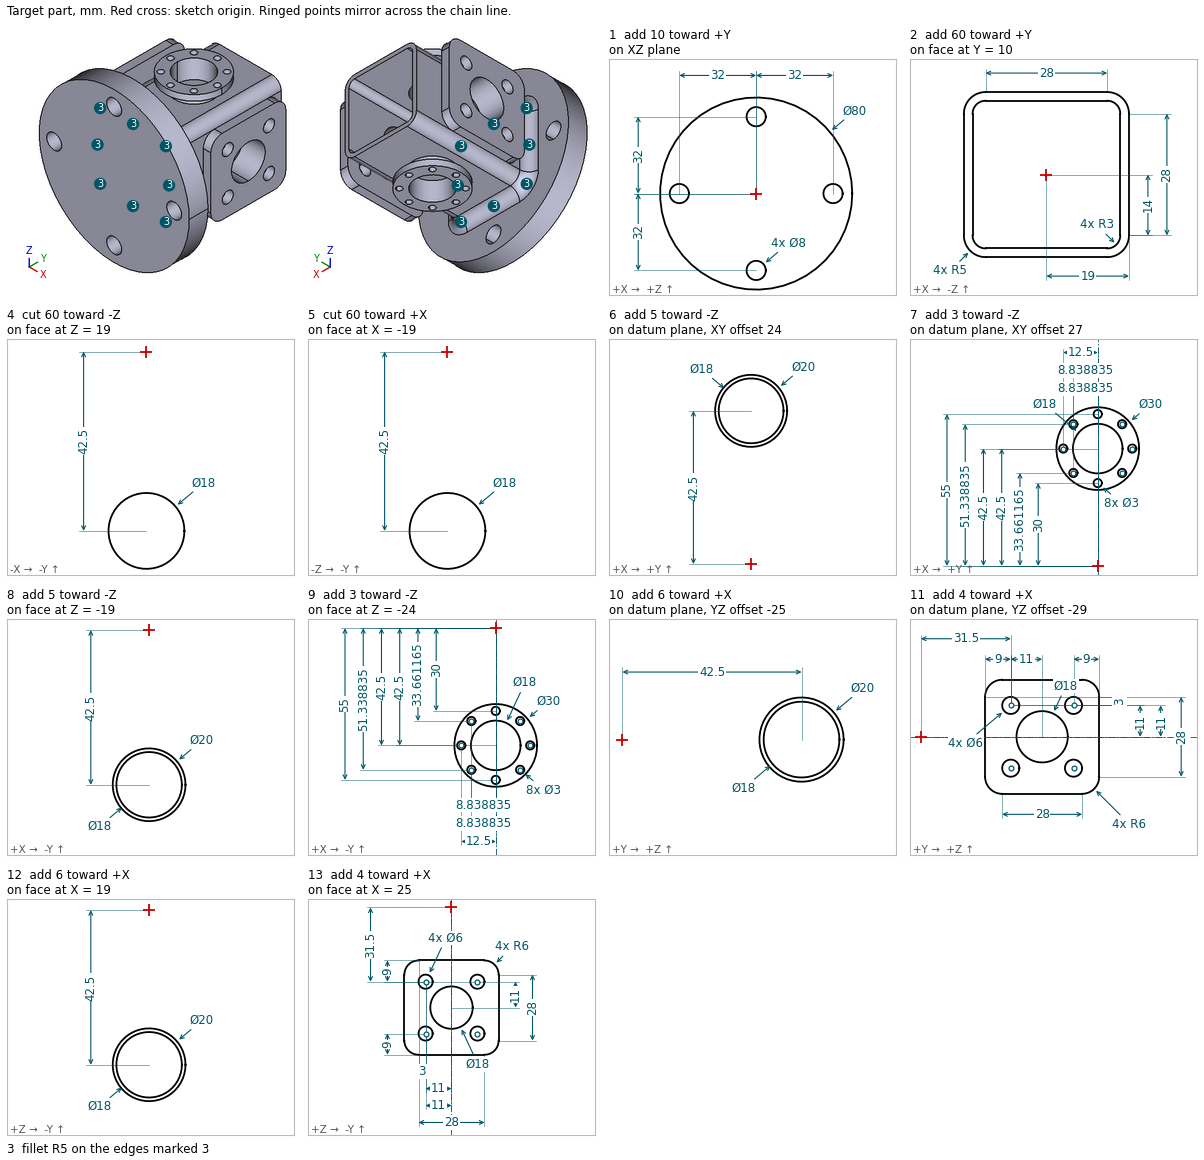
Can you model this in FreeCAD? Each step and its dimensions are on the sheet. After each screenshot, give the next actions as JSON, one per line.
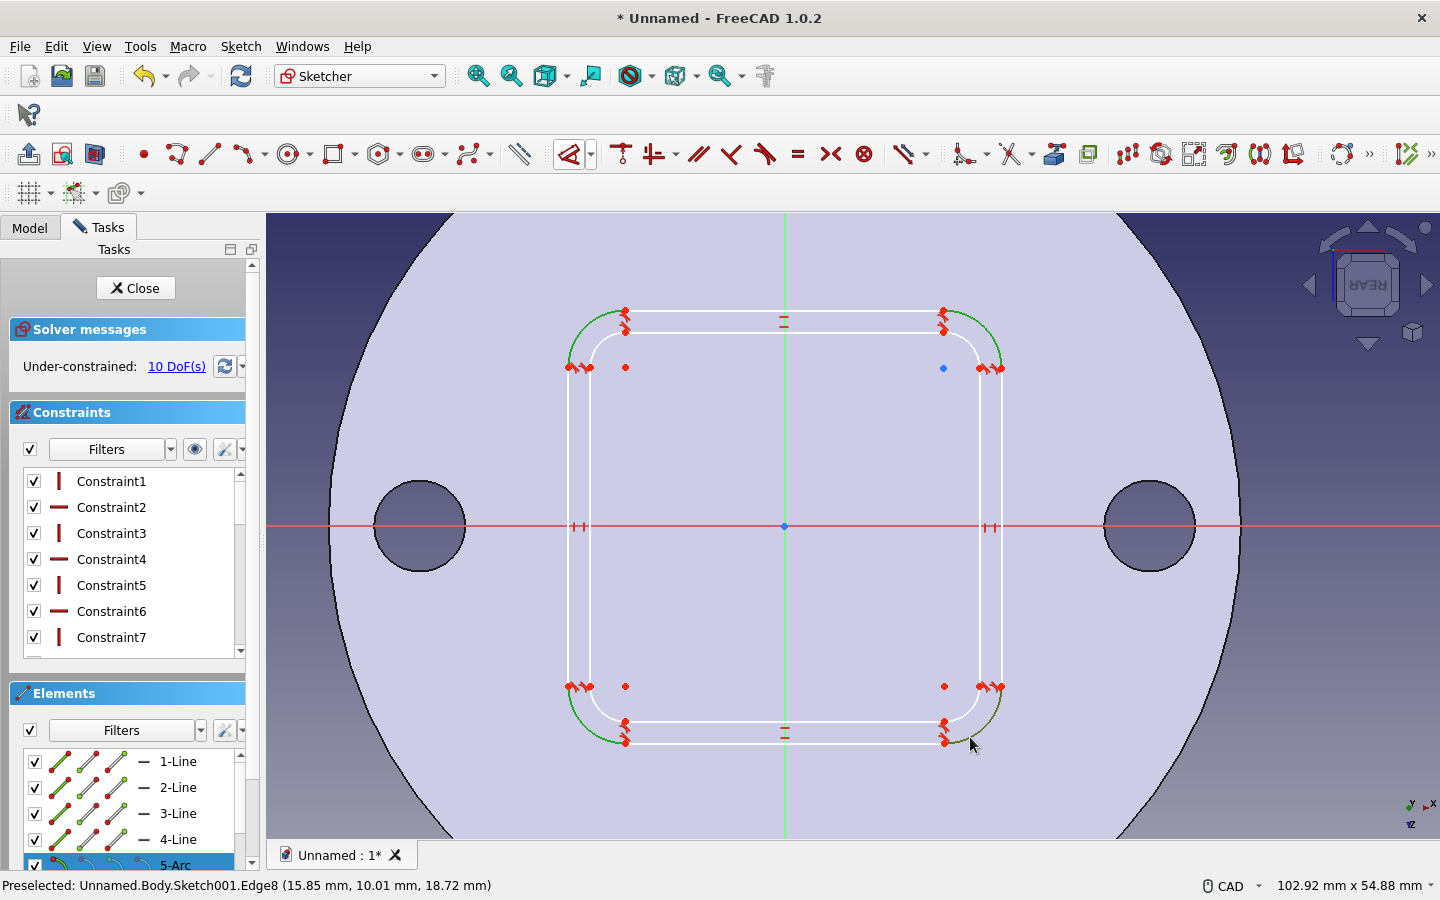
{"action": "key", "text": "e"}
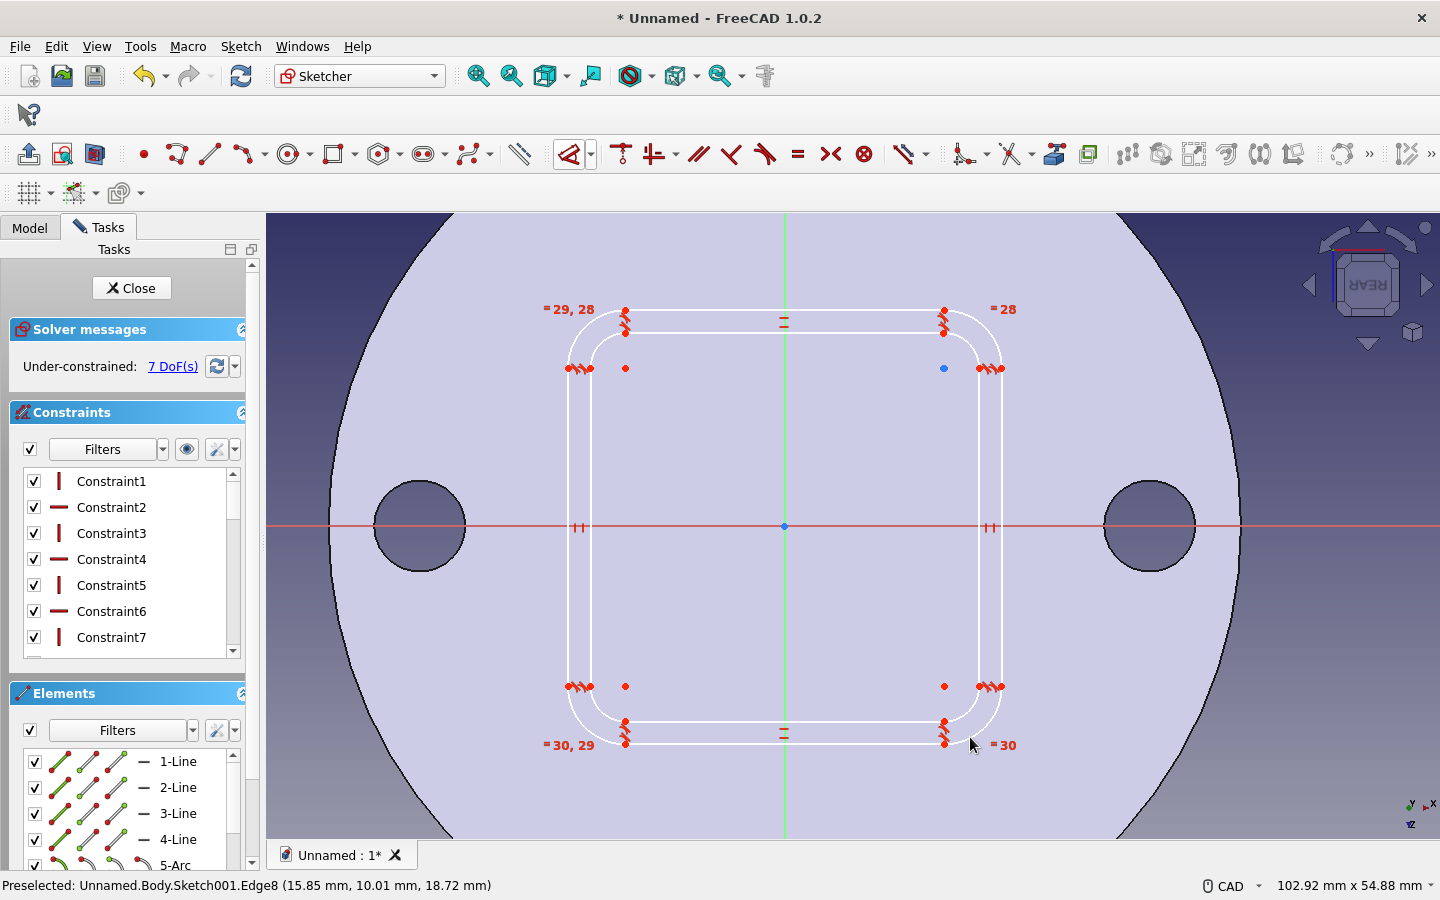
{"action": "left_click", "coordinate": [960, 718]}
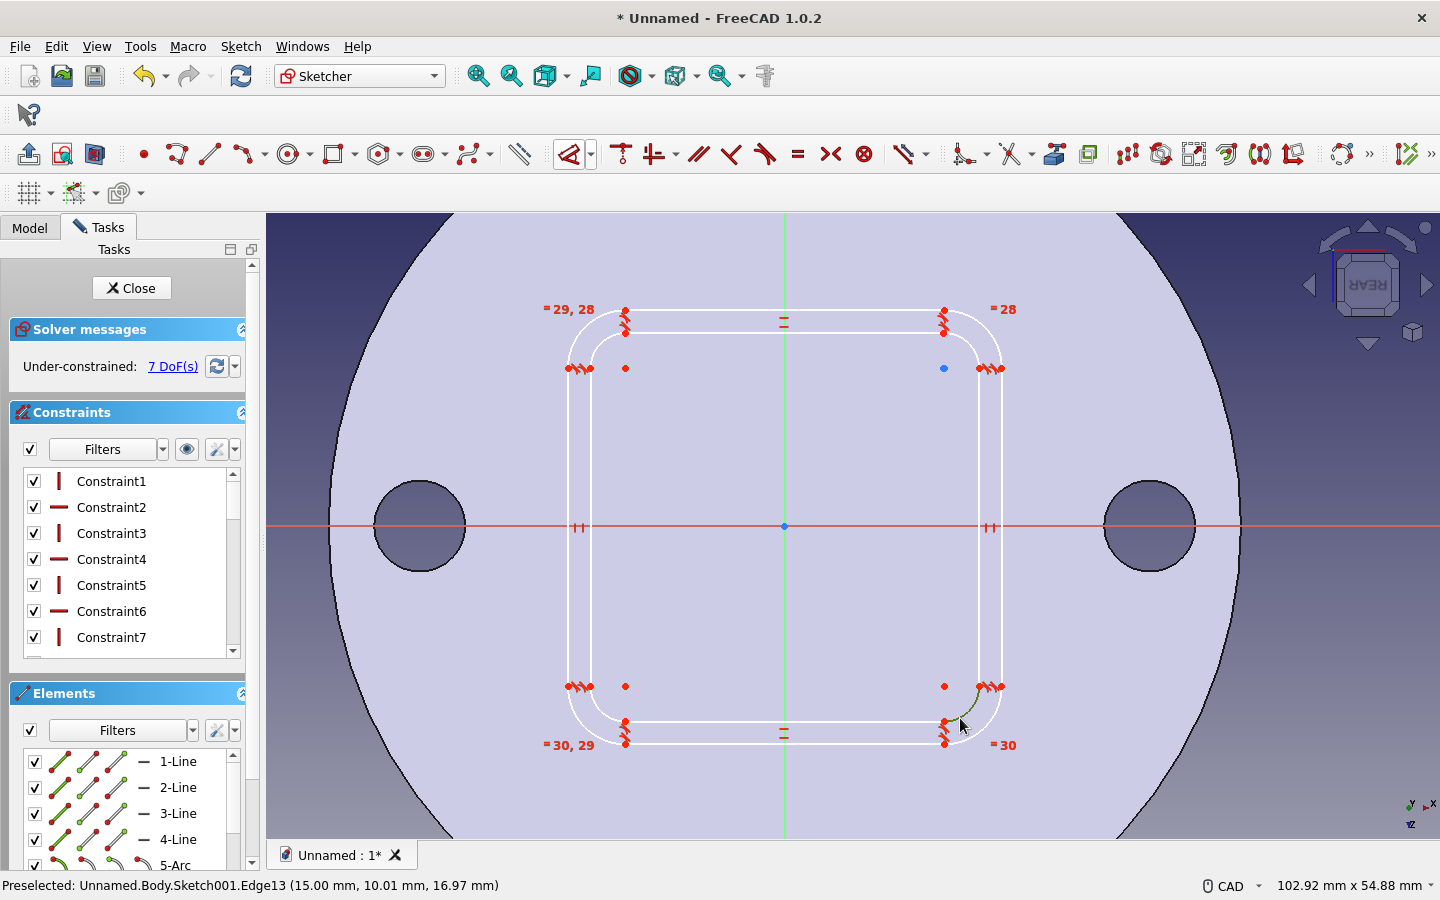
{"action": "left_click", "coordinate": [975, 352]}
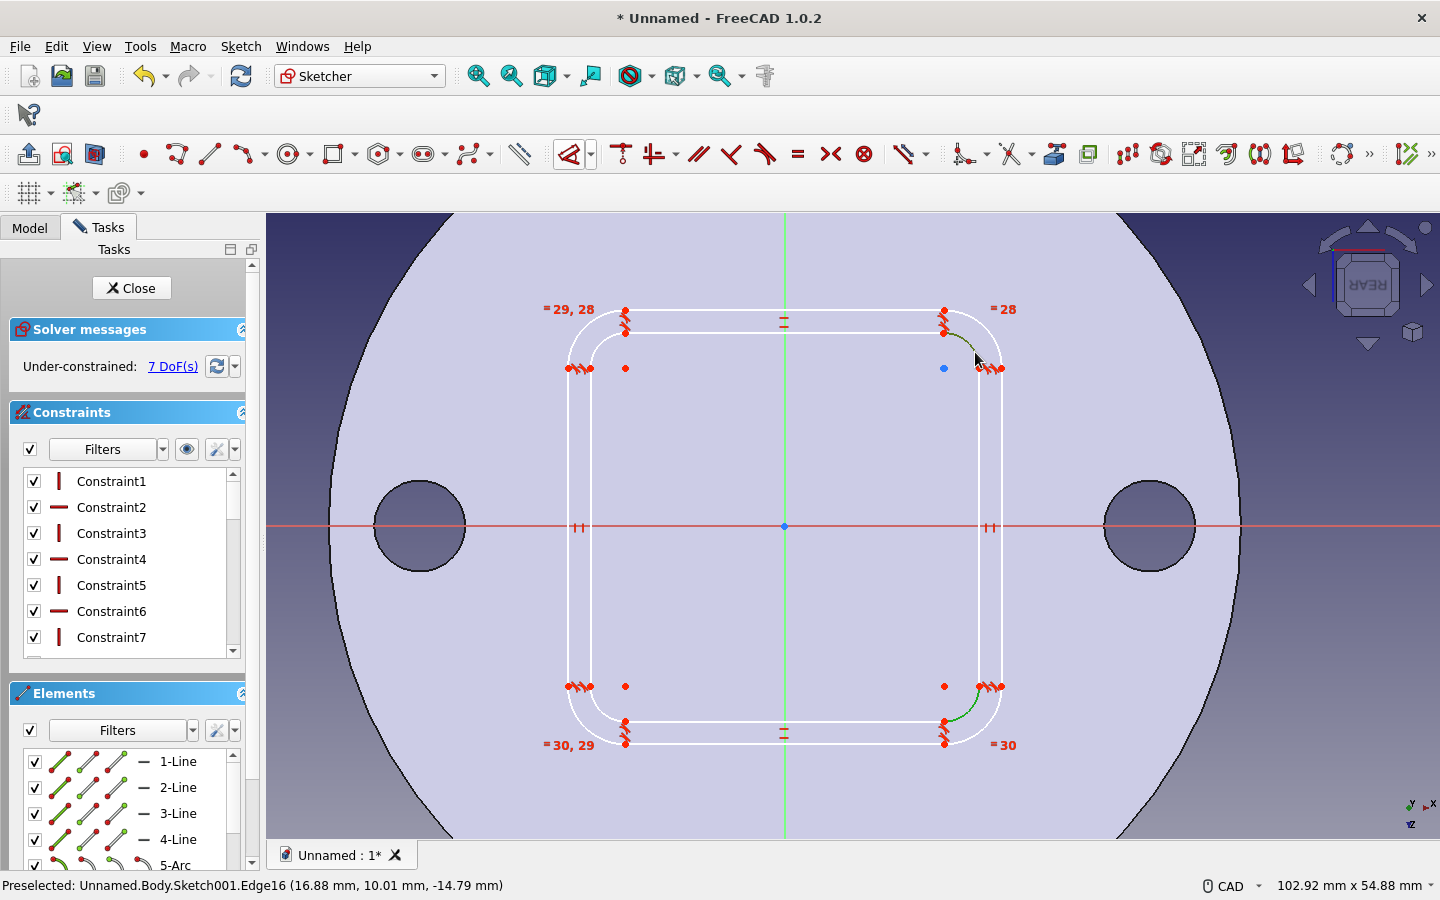
{"action": "key", "text": "e"}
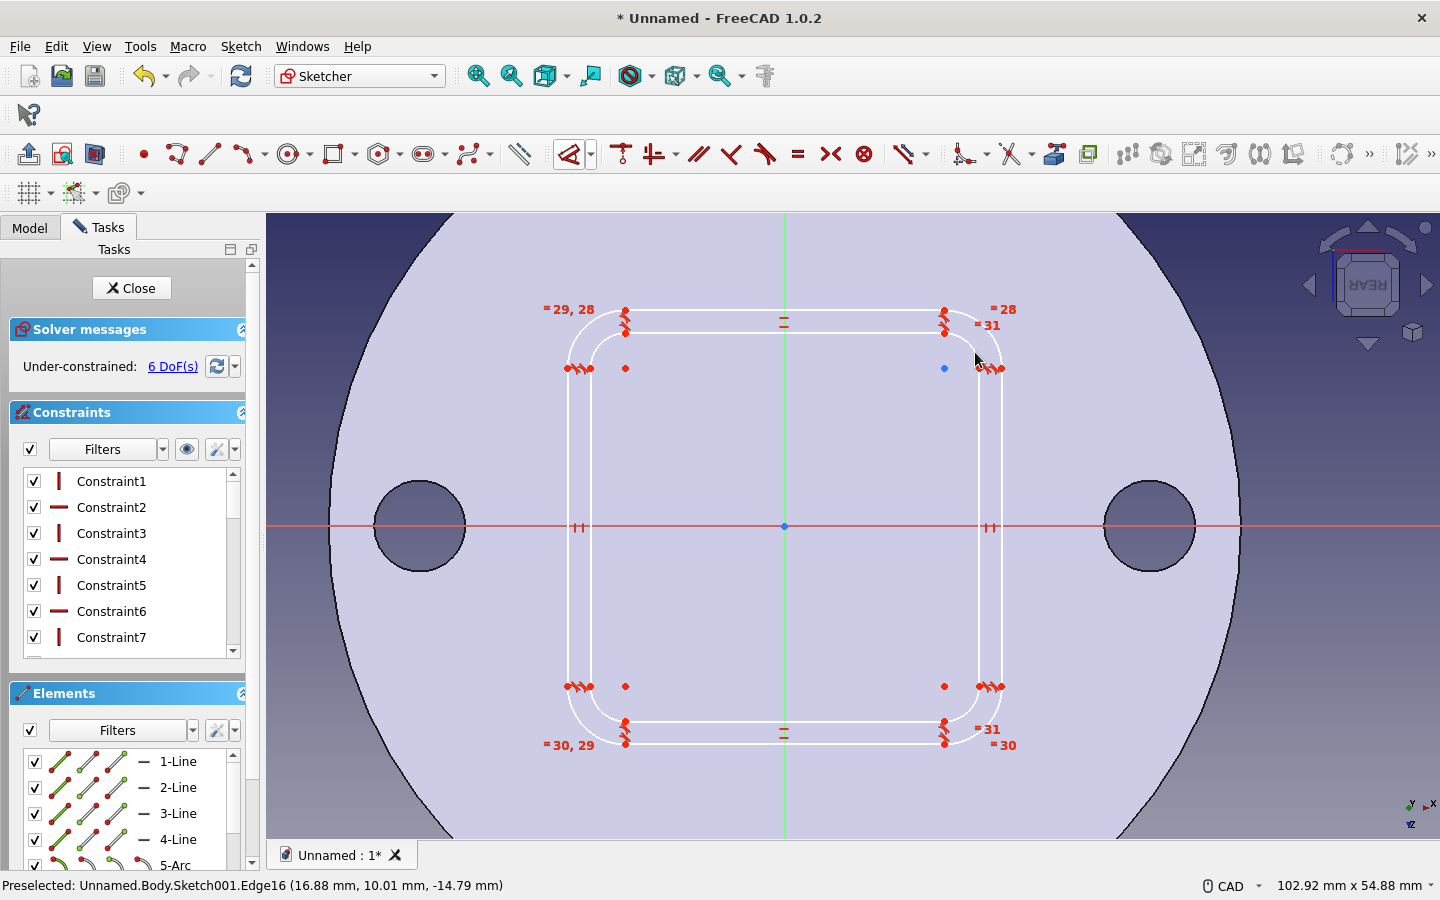
{"action": "left_click", "coordinate": [996, 342]}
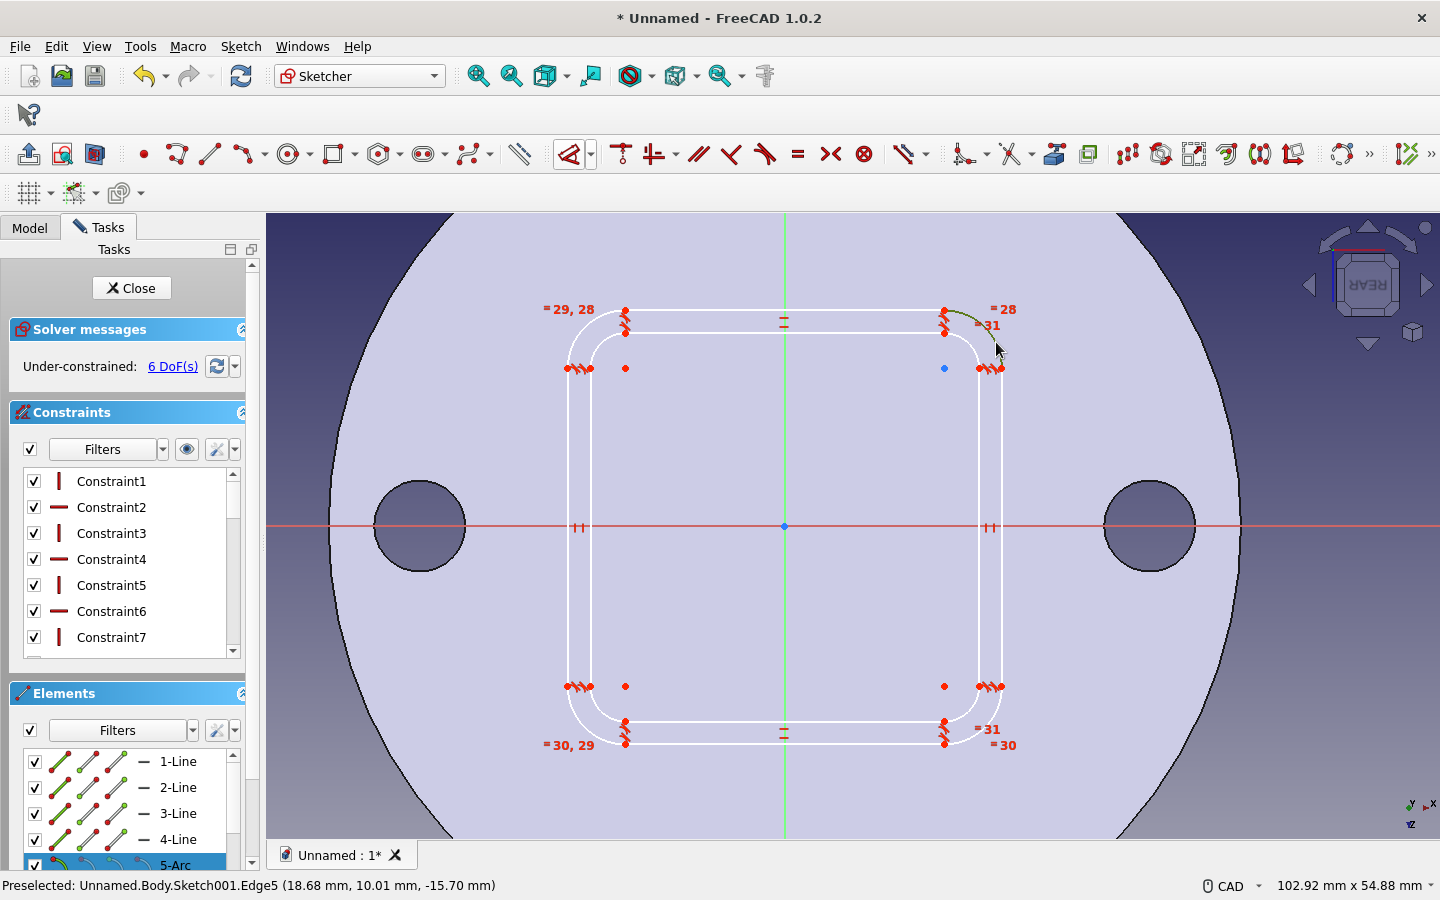
{"action": "key", "text": "k r"}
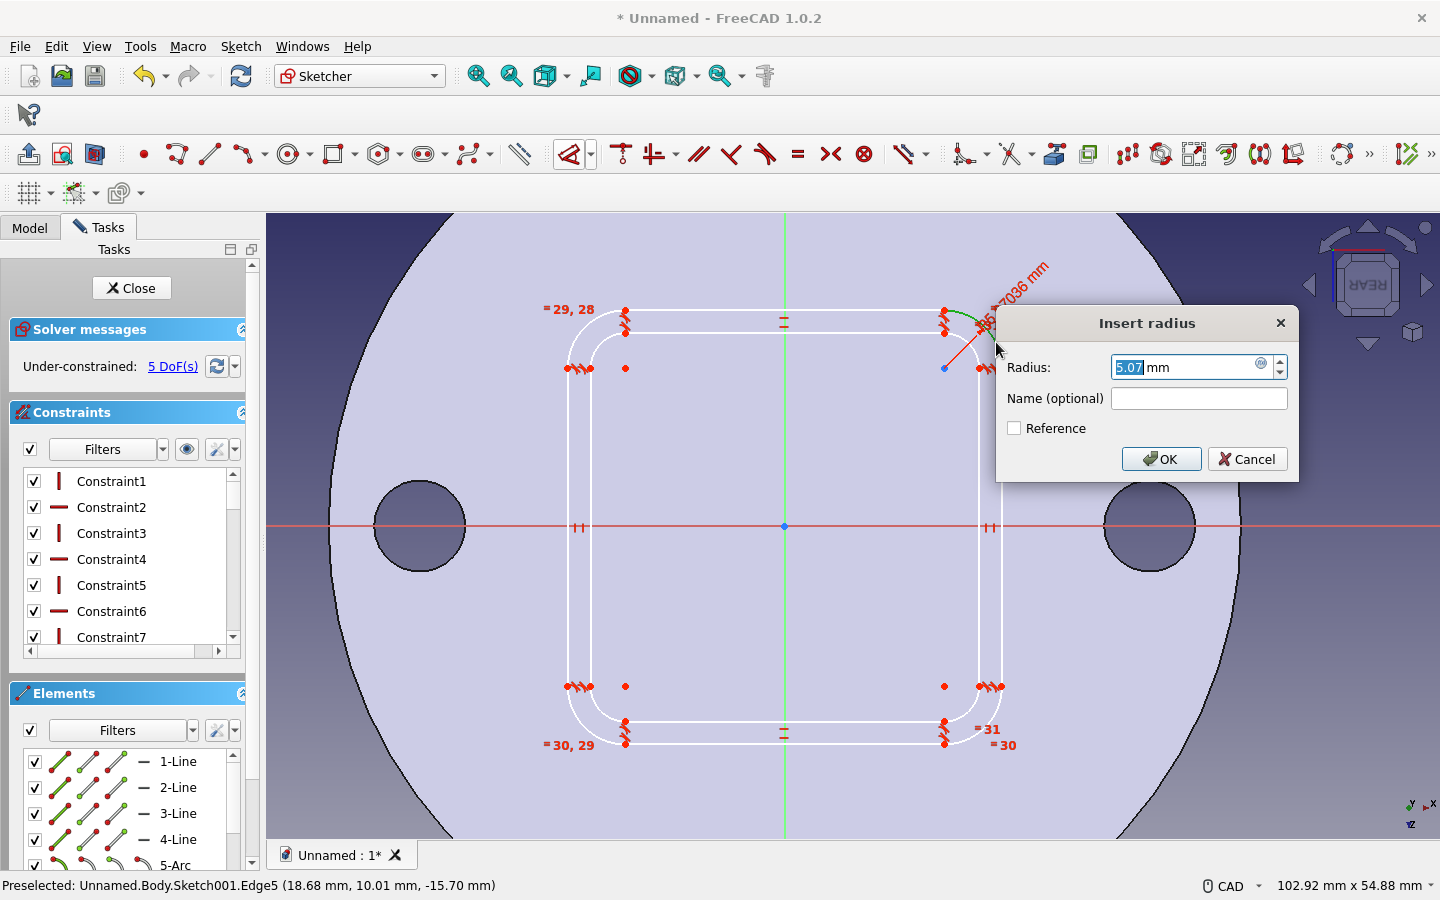
{"action": "type", "text": "5"}
{"action": "key", "text": "Return"}